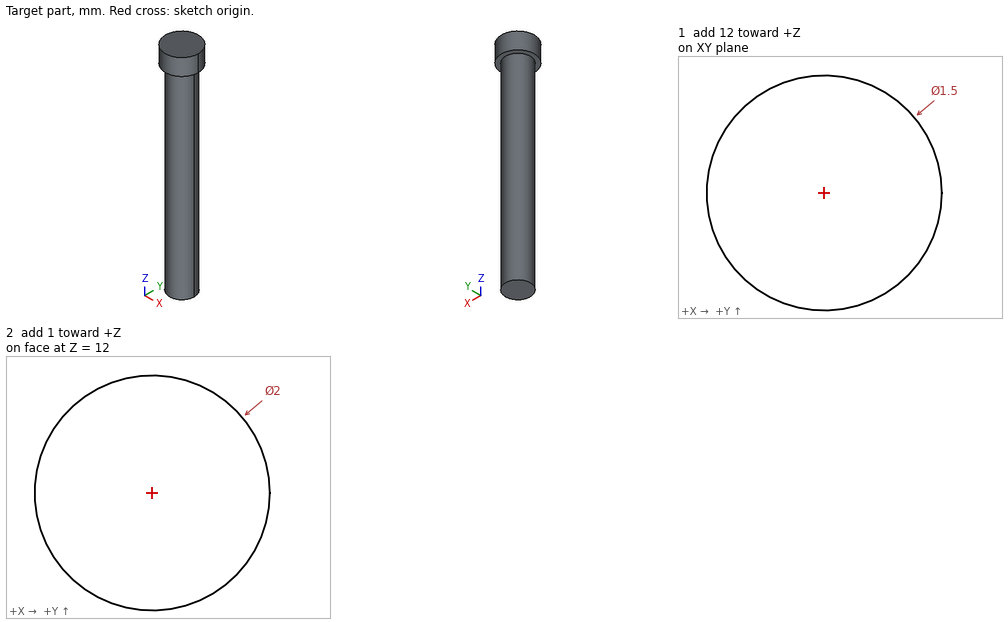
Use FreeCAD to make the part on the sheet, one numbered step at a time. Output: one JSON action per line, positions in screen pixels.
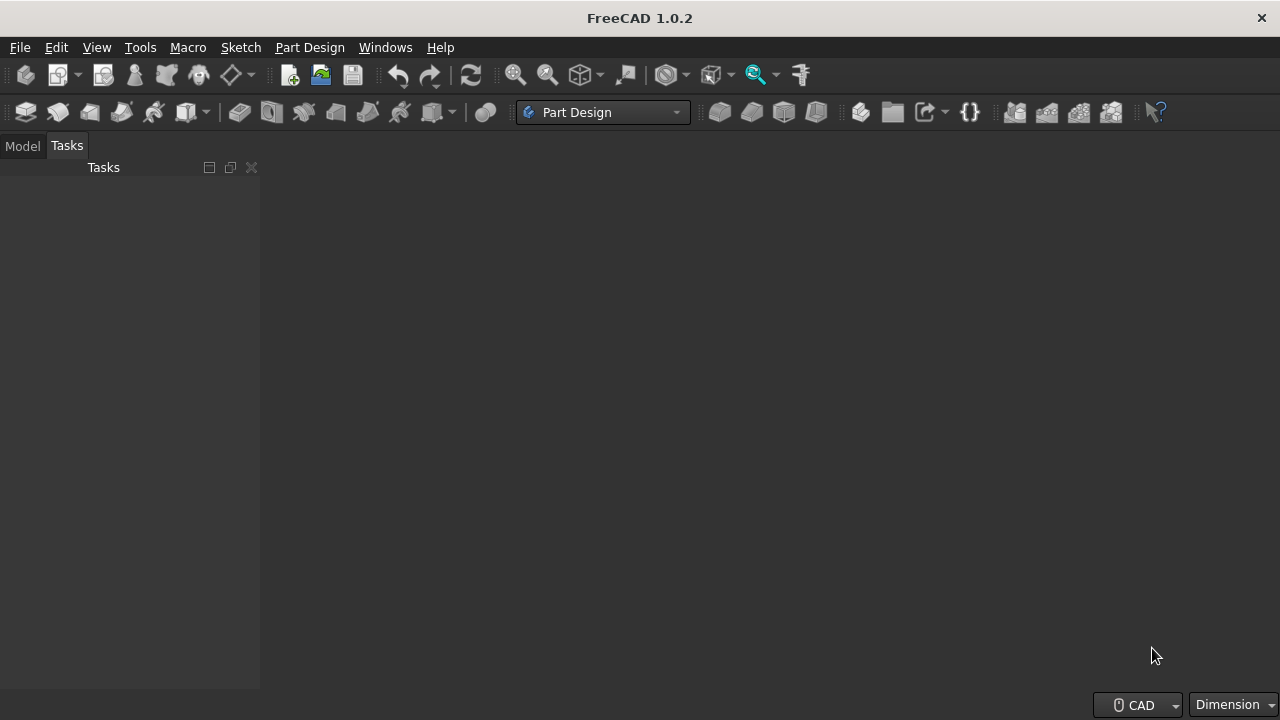
{"action": "left_click", "coordinate": [290, 76]}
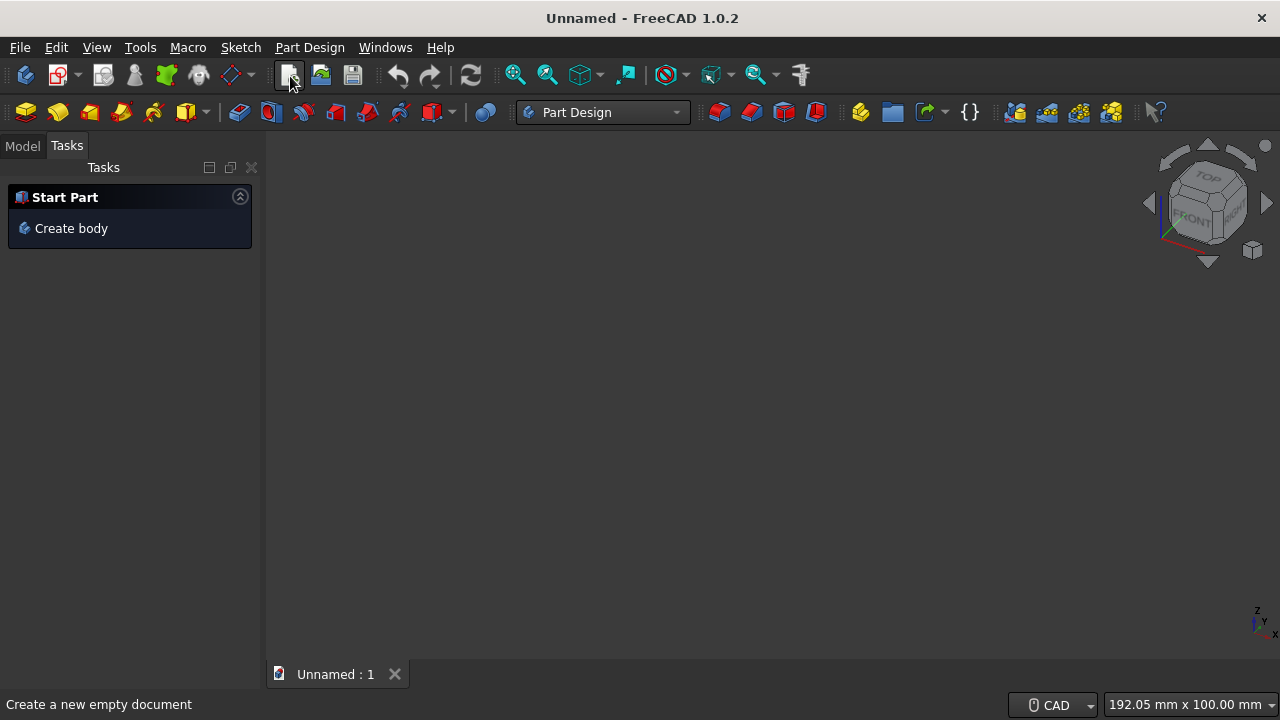
{"action": "left_click", "coordinate": [58, 76]}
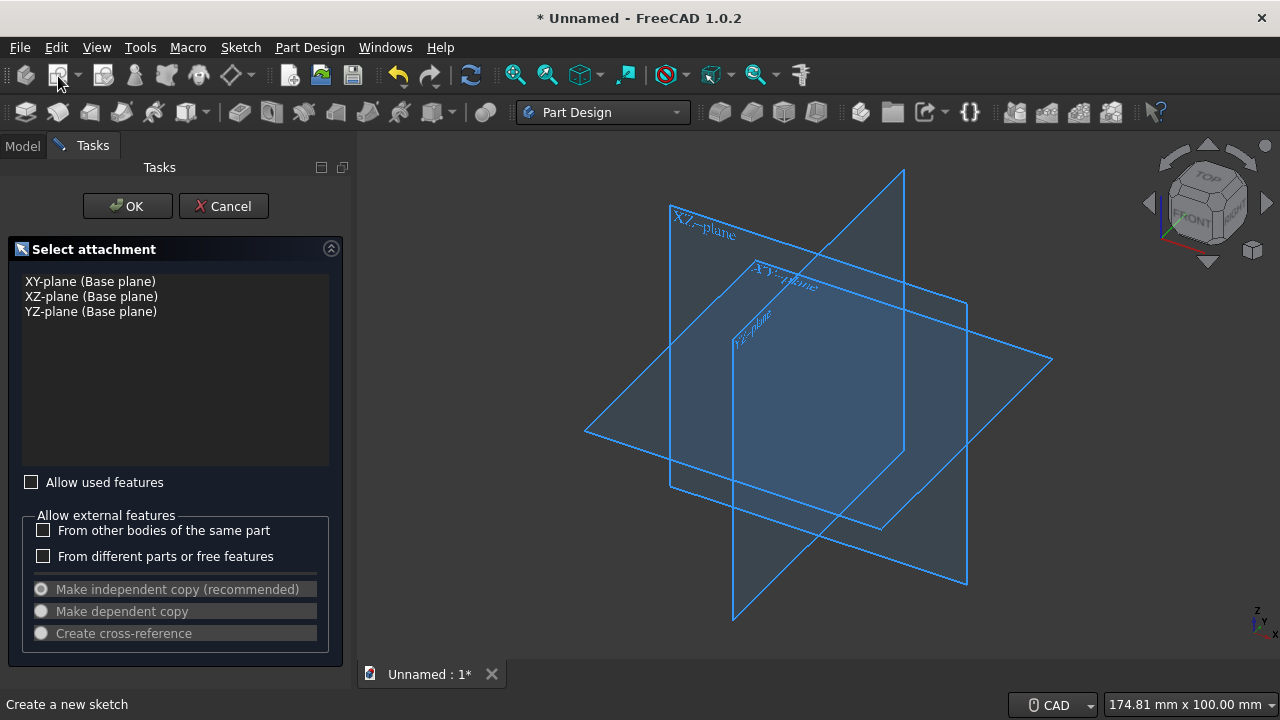
{"action": "left_click", "coordinate": [82, 282]}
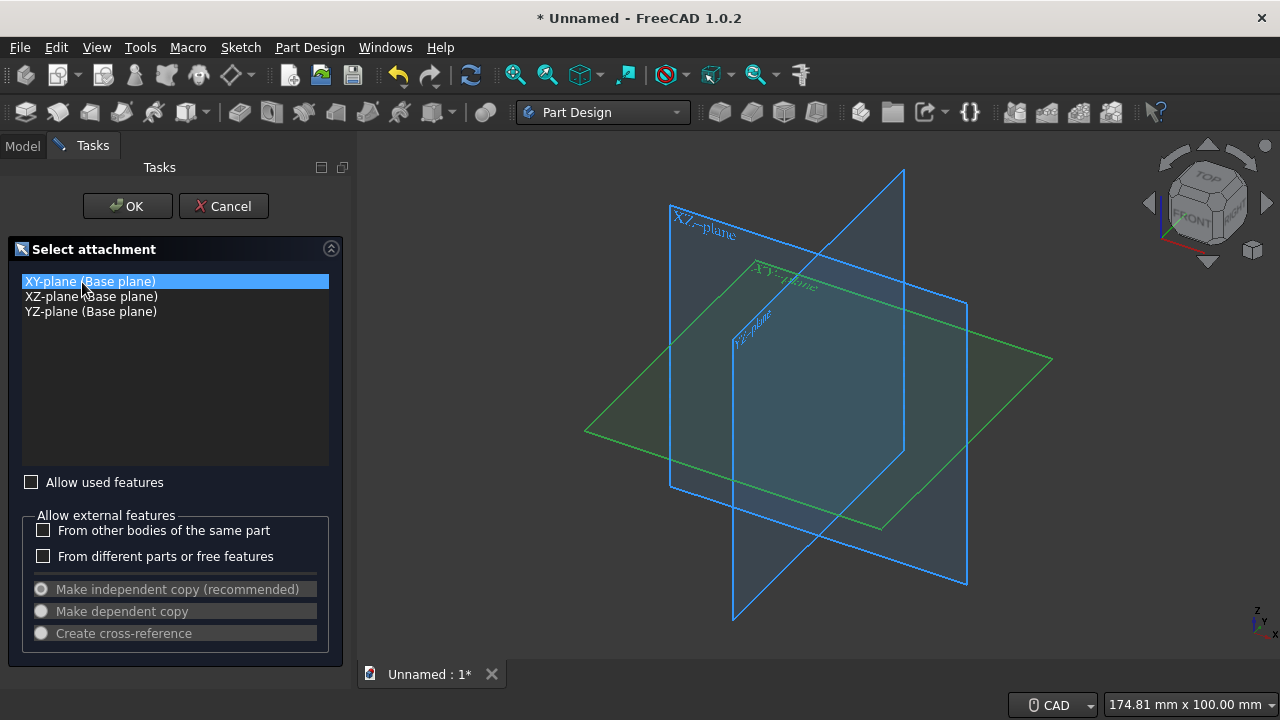
{"action": "left_click", "coordinate": [128, 206]}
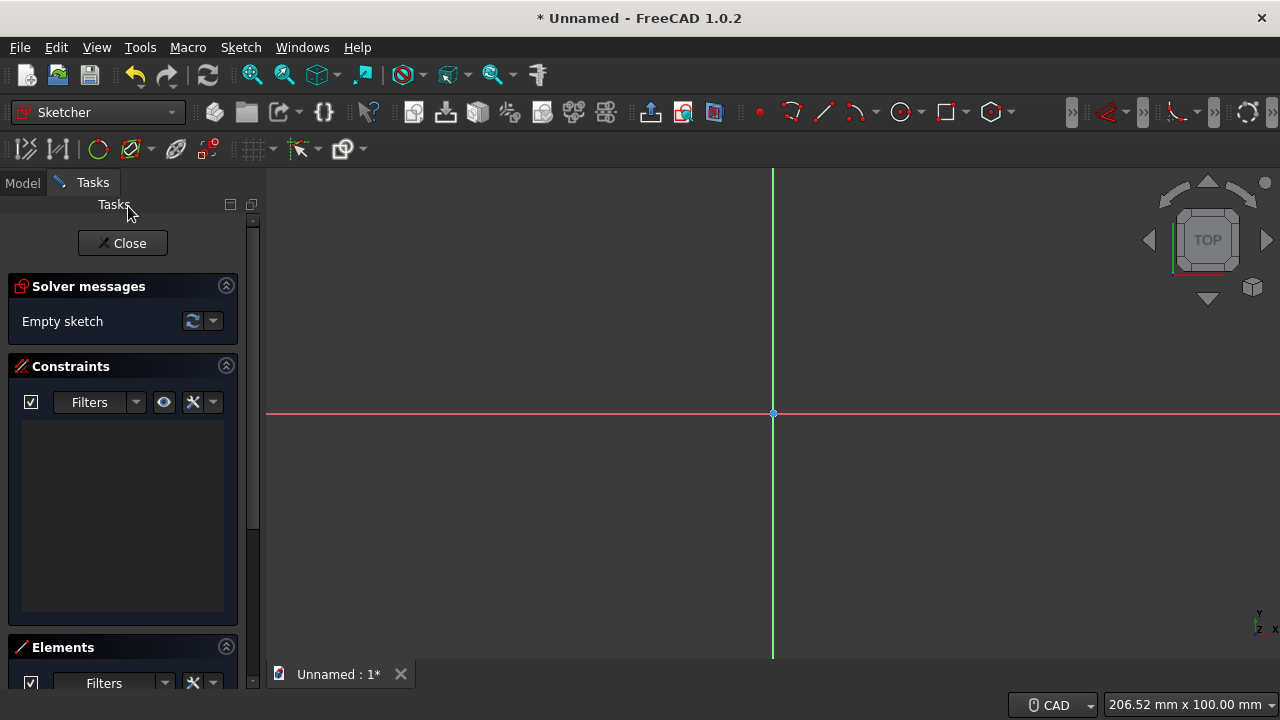
{"action": "scroll", "coordinate": [777, 414], "scroll_direction": "up", "scroll_amount": 15}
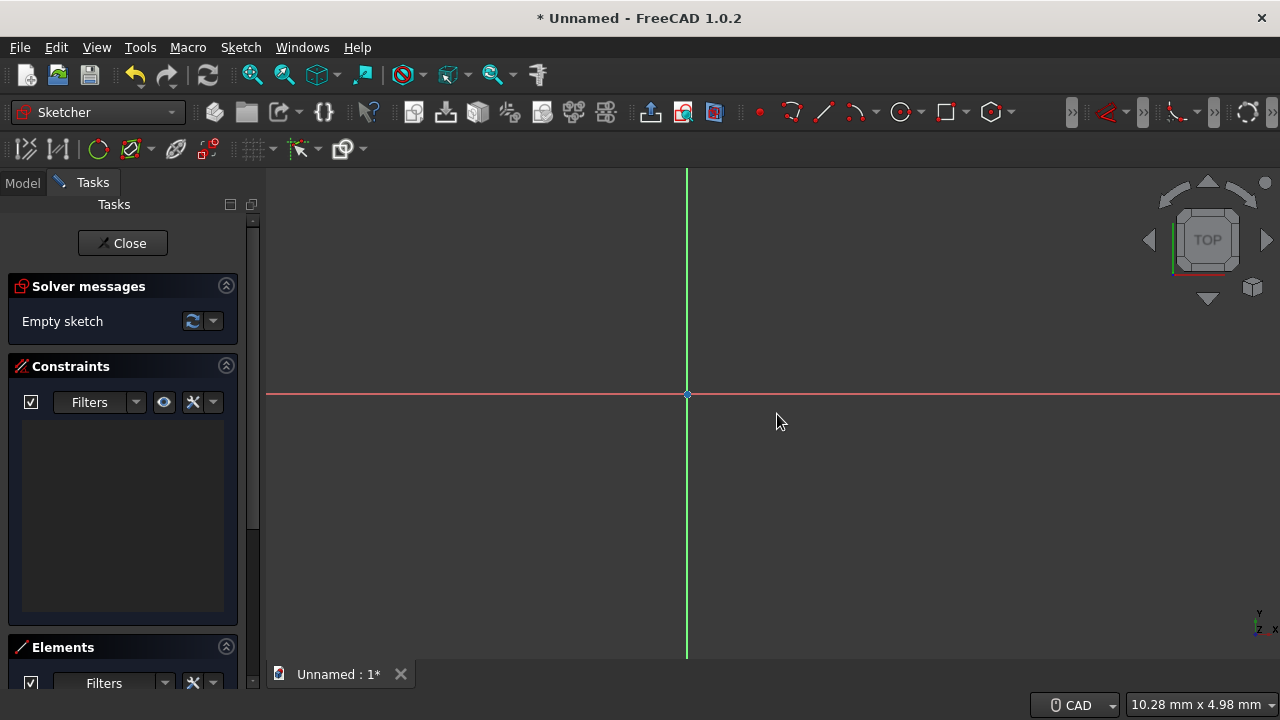
{"action": "scroll", "coordinate": [673, 379], "scroll_direction": "up", "scroll_amount": 4}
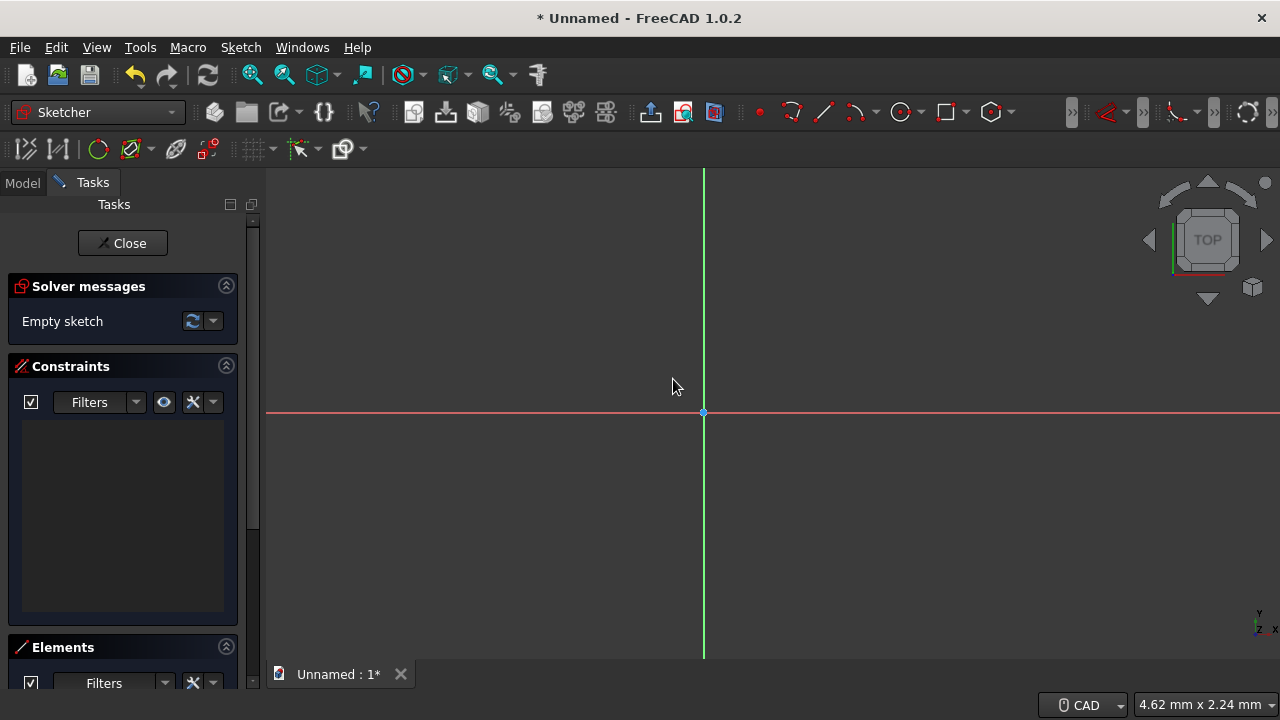
{"action": "left_click", "coordinate": [902, 112]}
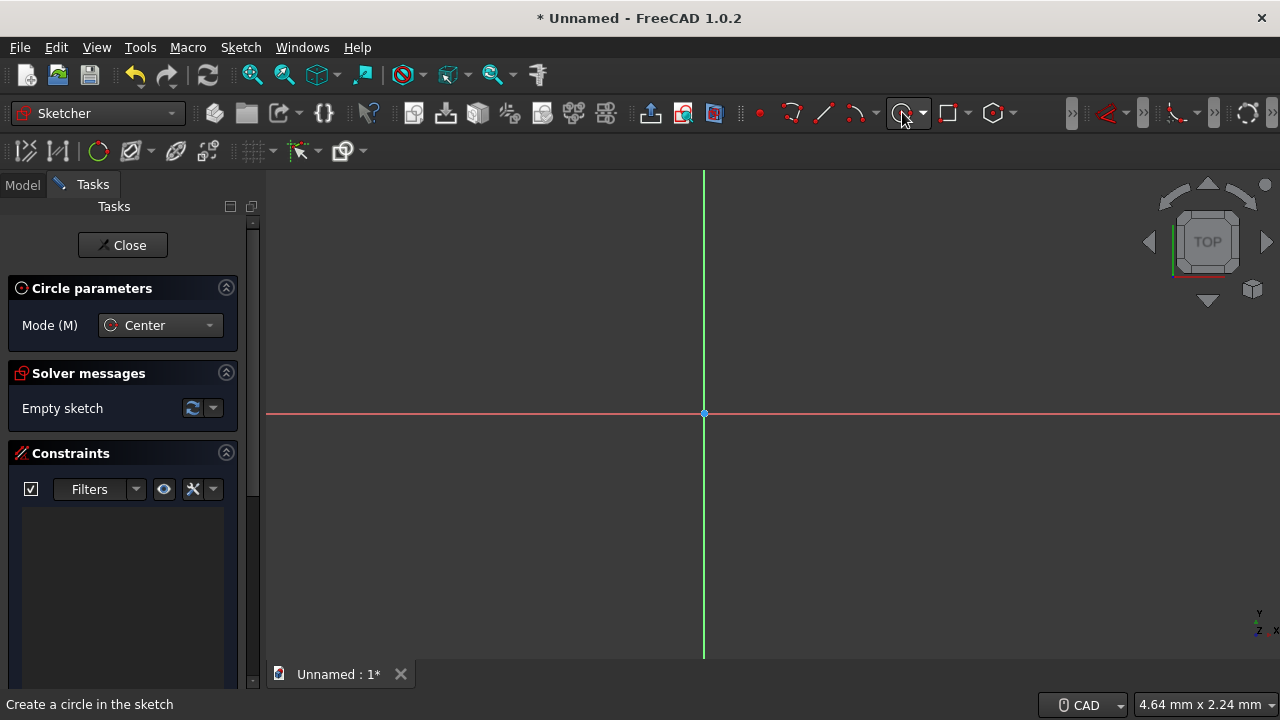
{"action": "left_click", "coordinate": [704, 414]}
{"action": "mouse_move", "coordinate": [820, 298]}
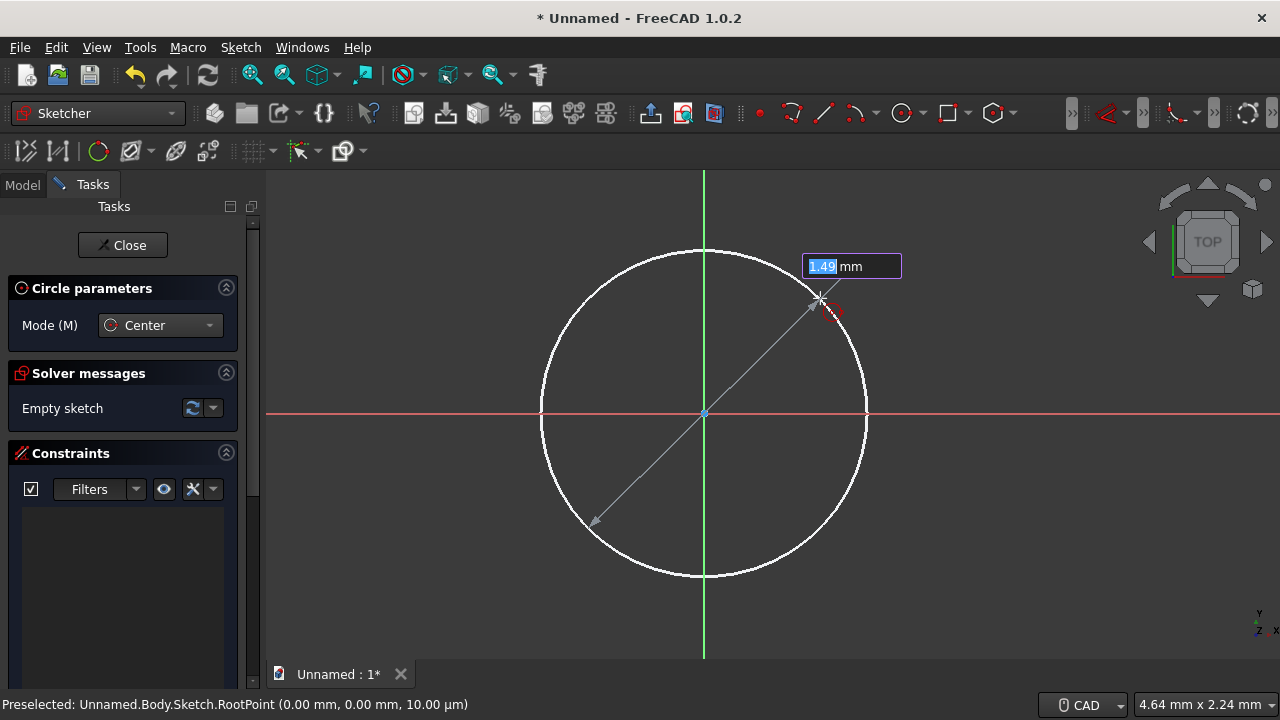
{"action": "type", "text": "1.5"}
{"action": "key", "text": "Return"}
{"action": "key", "text": "Escape"}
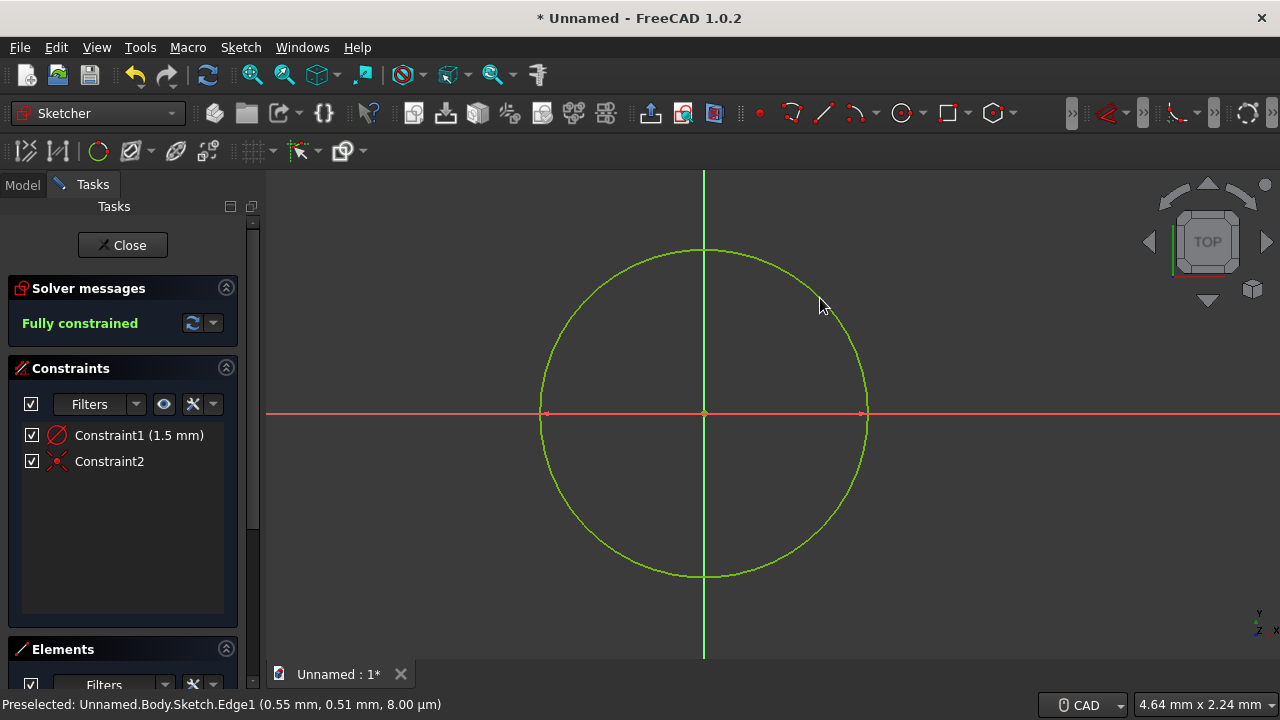
{"action": "left_click", "coordinate": [123, 245]}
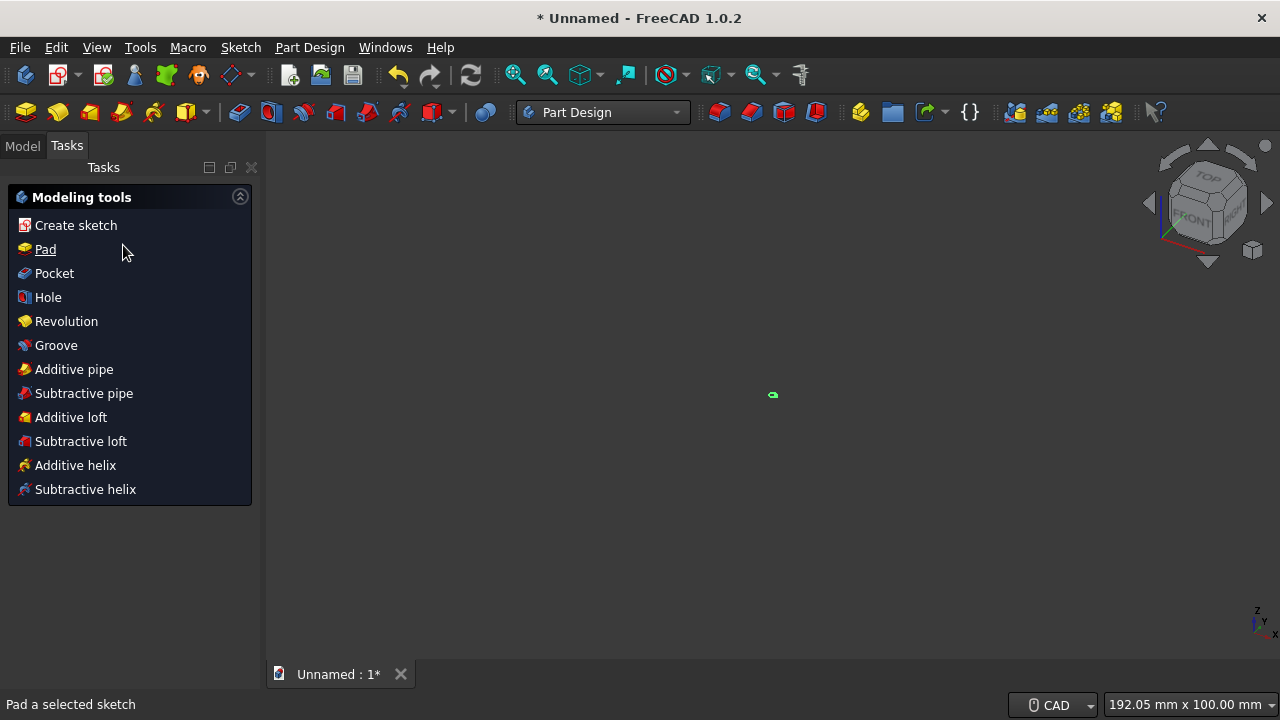
{"action": "left_click", "coordinate": [26, 112]}